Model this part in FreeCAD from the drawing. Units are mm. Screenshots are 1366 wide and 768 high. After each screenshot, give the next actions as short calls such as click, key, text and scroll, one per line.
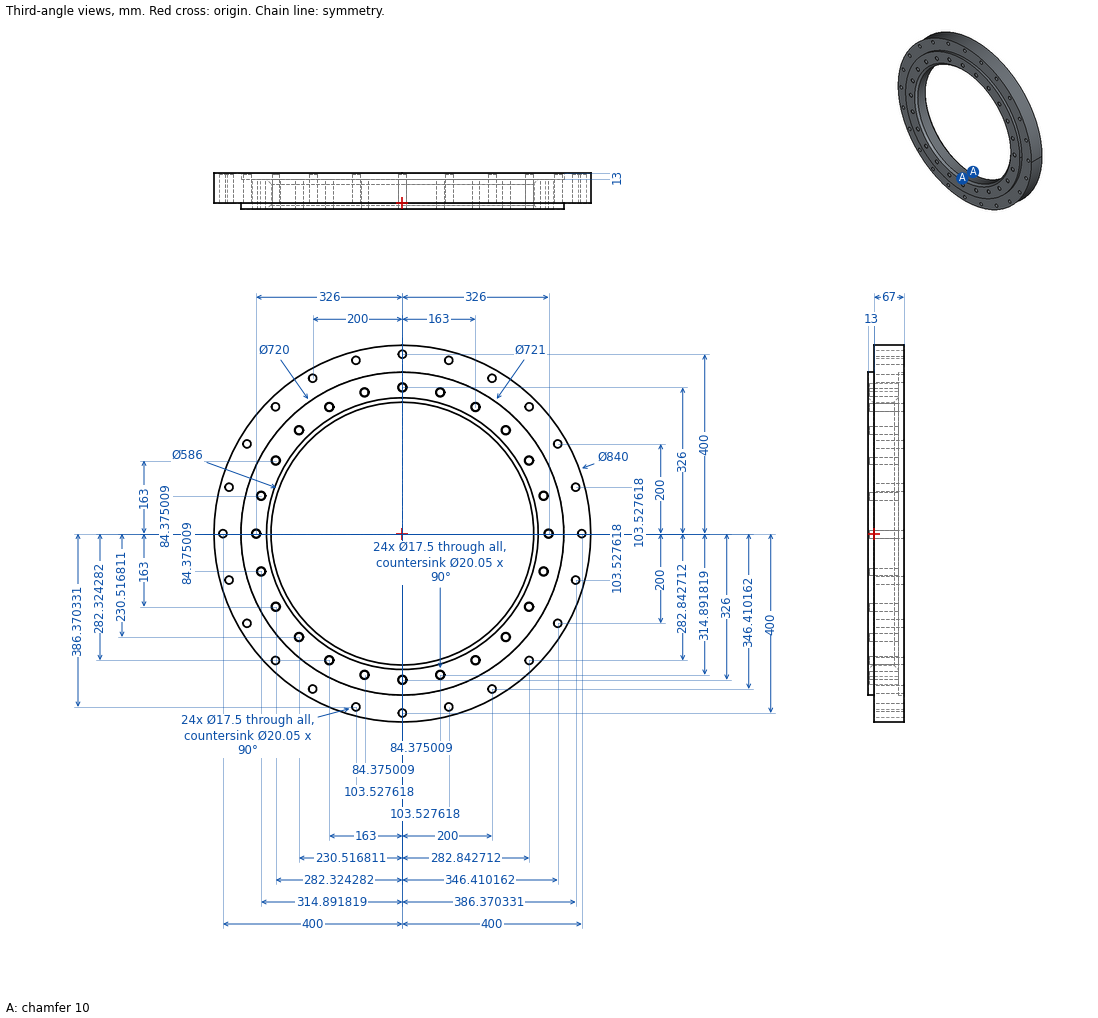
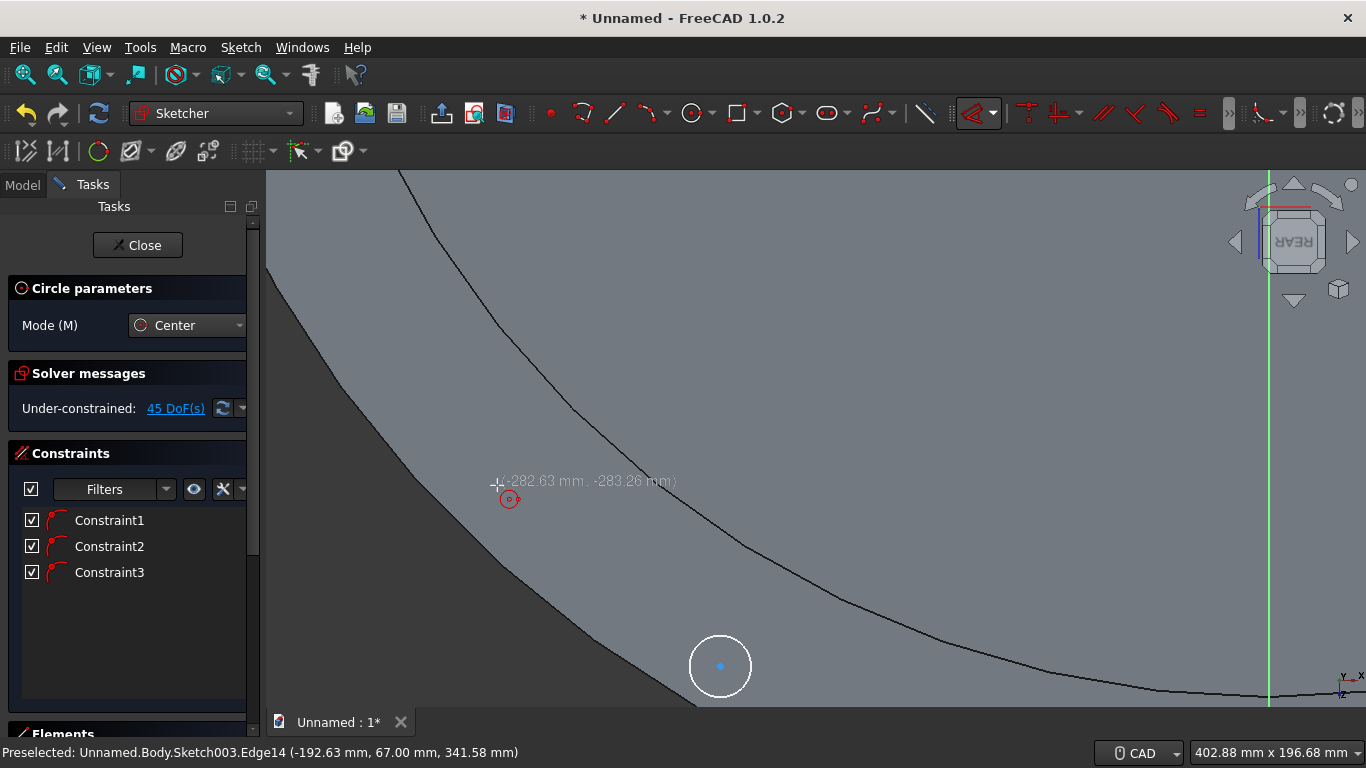
scroll(644, 582, down, 9)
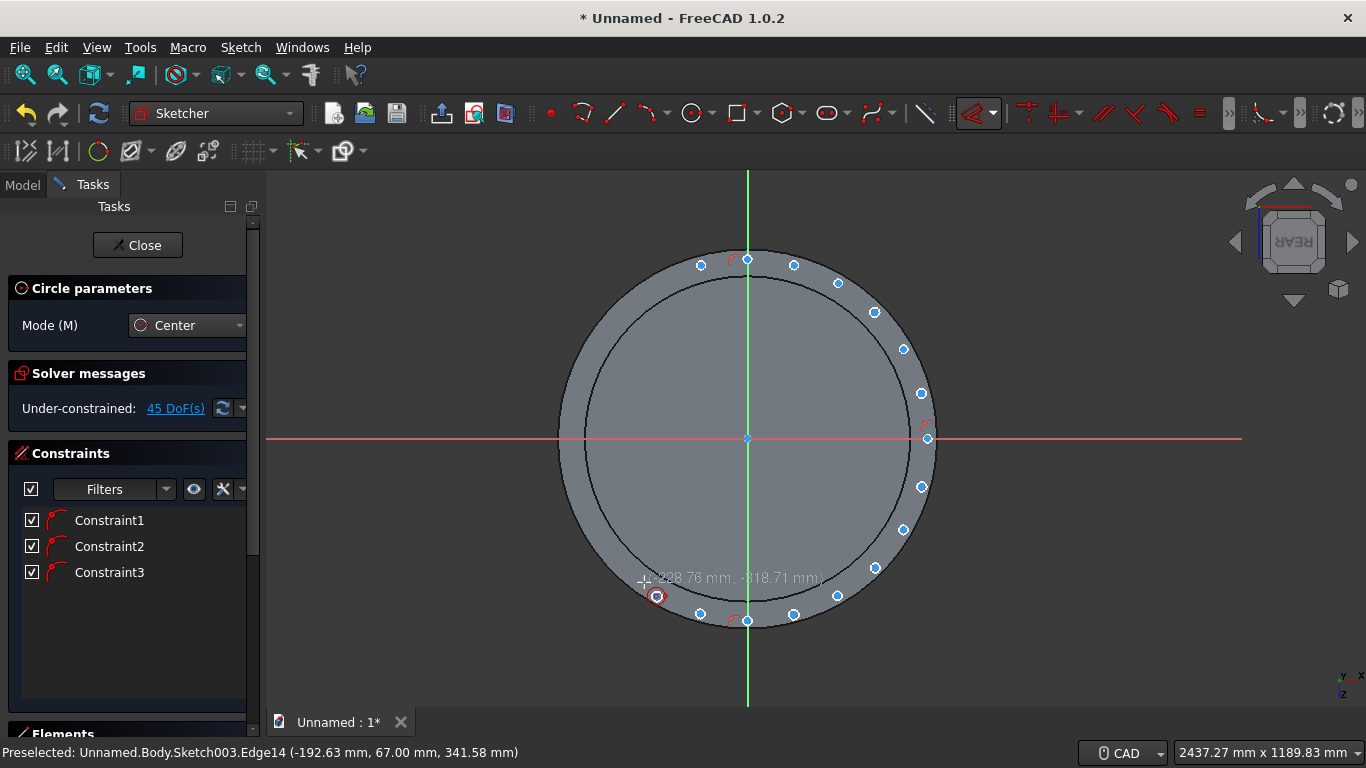
click(620, 567)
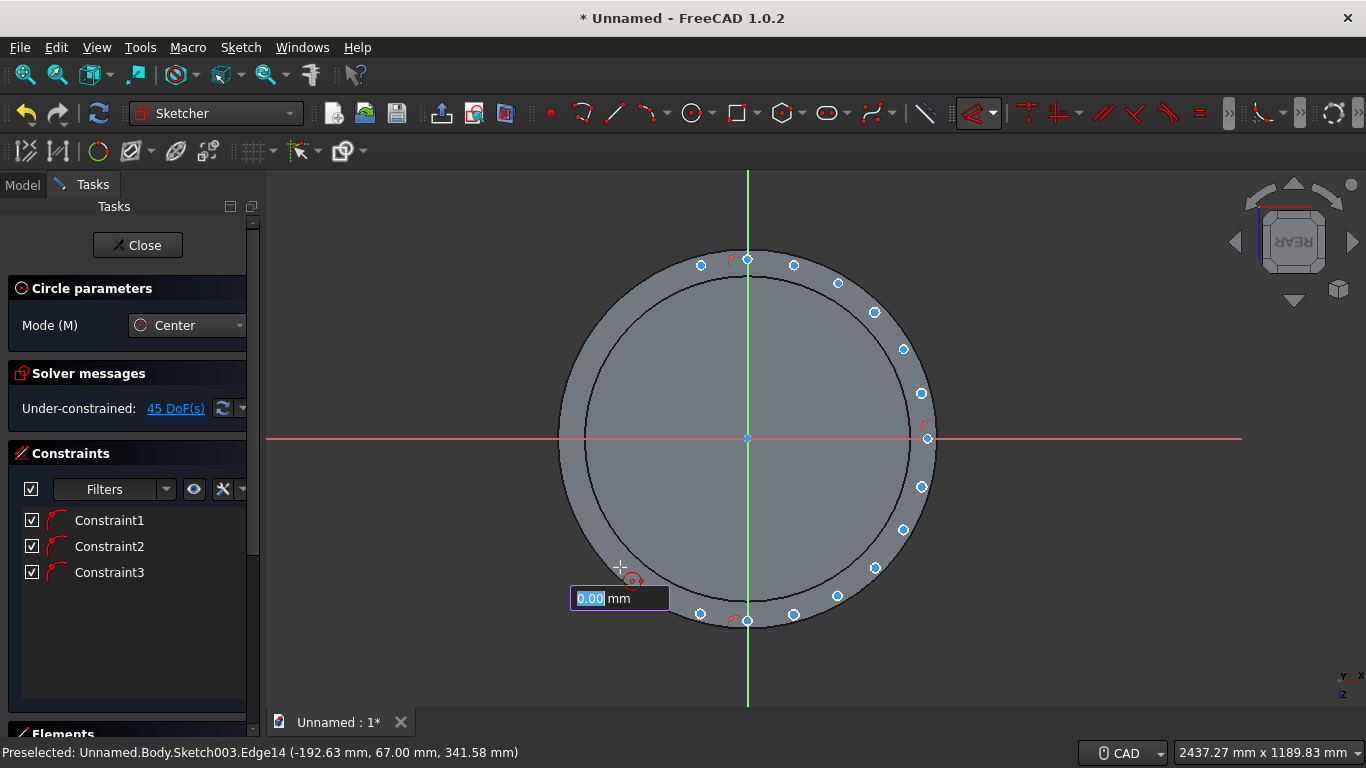
scroll(623, 564, up, 7)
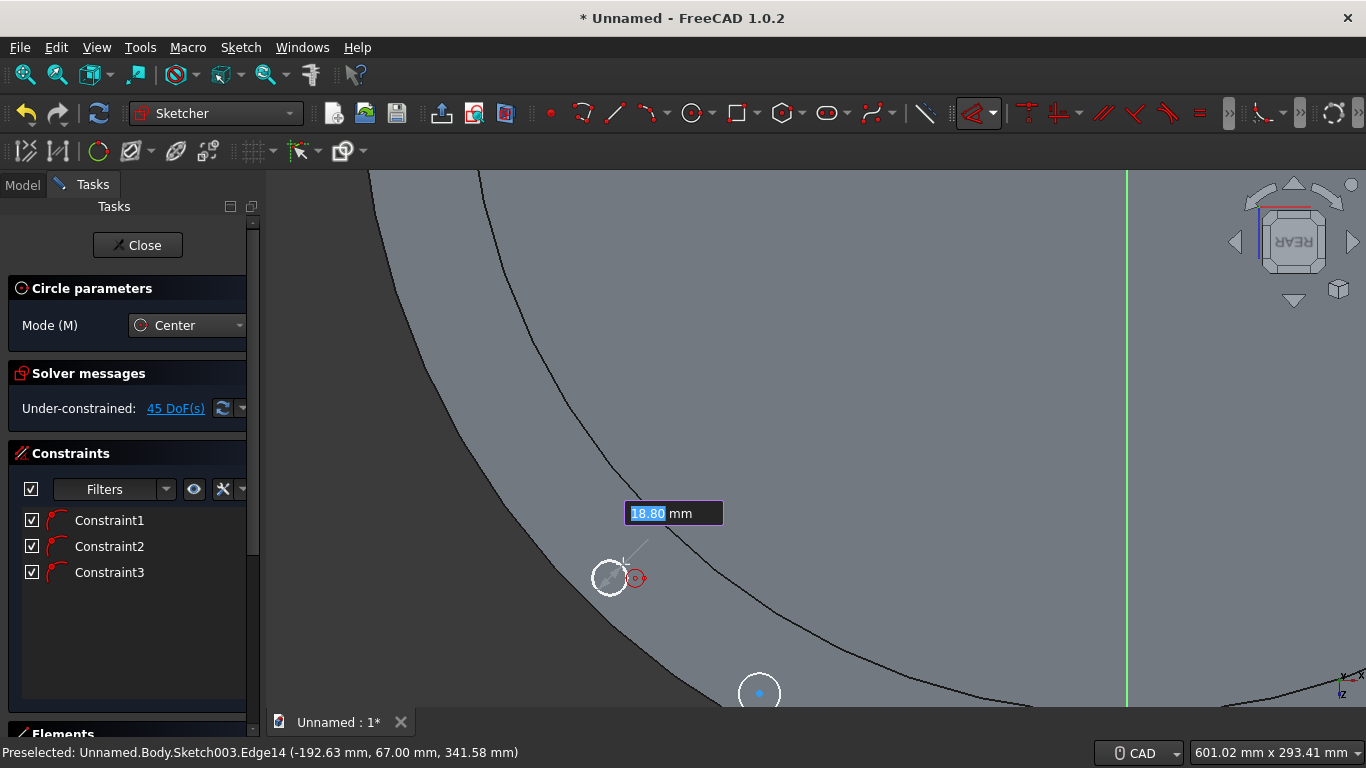
click(621, 561)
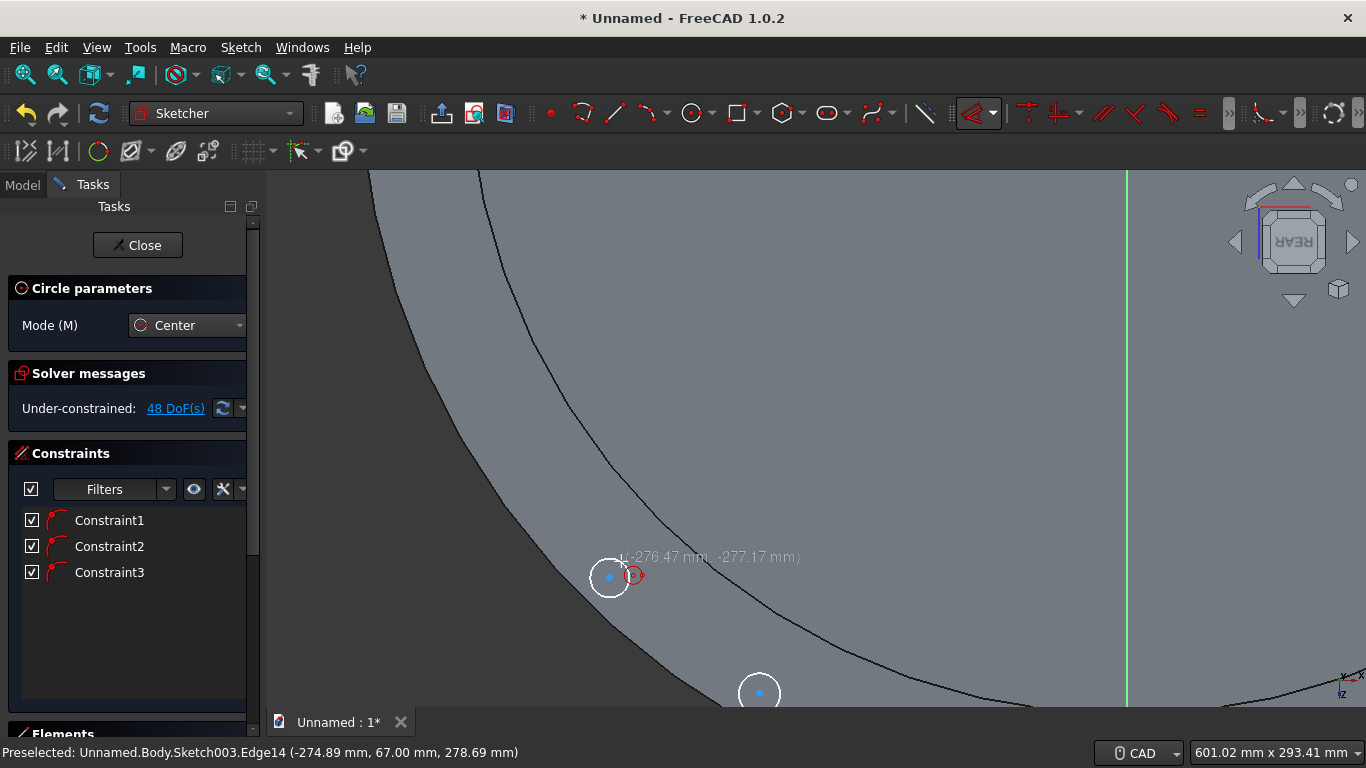
scroll(493, 421, up, 2)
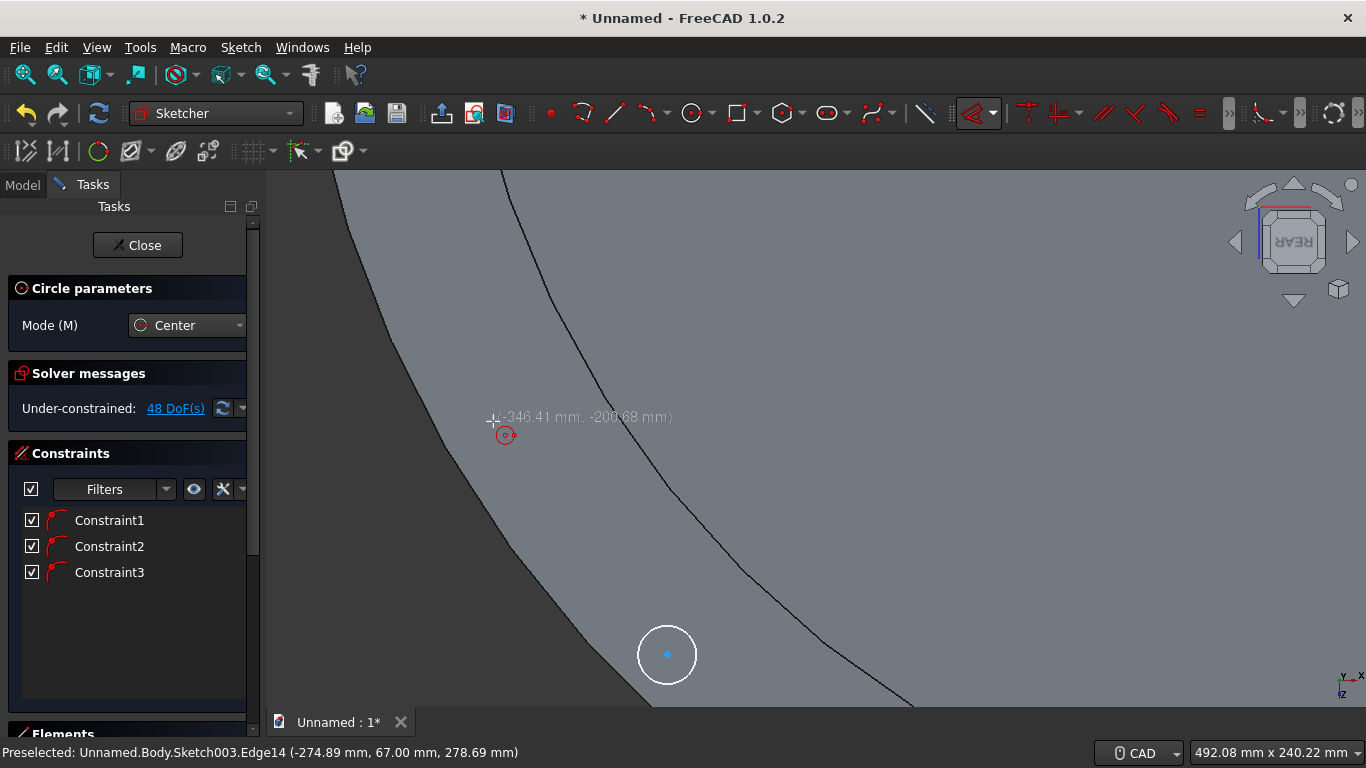
scroll(611, 550, down, 9)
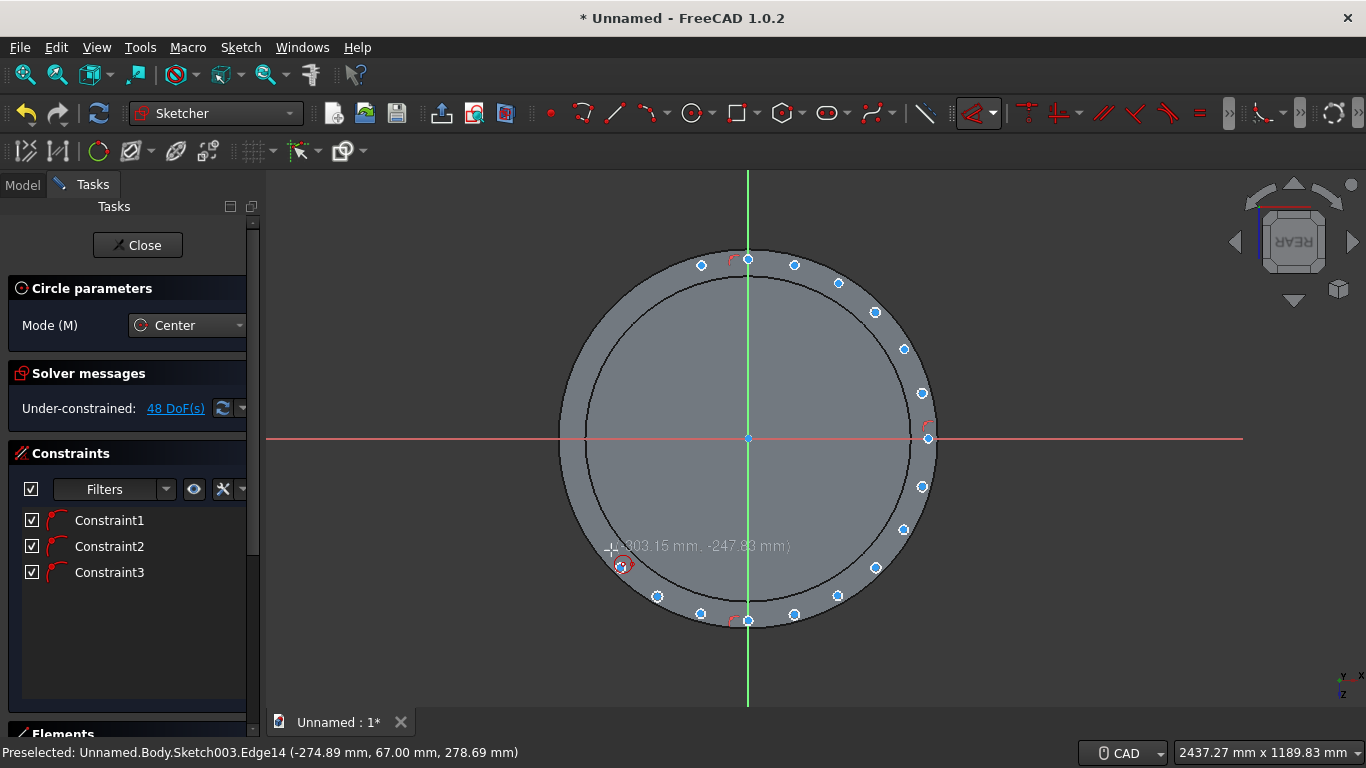
click(592, 529)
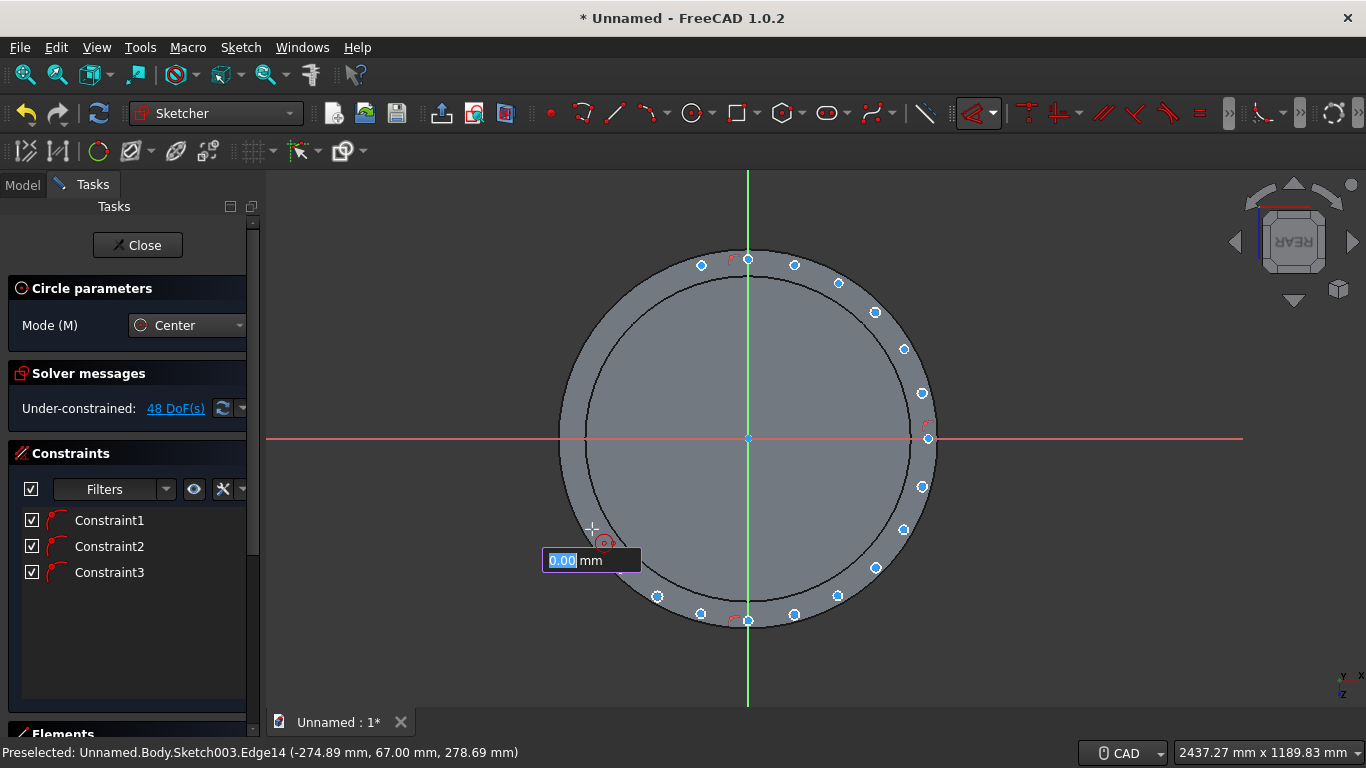
scroll(595, 526, up, 7)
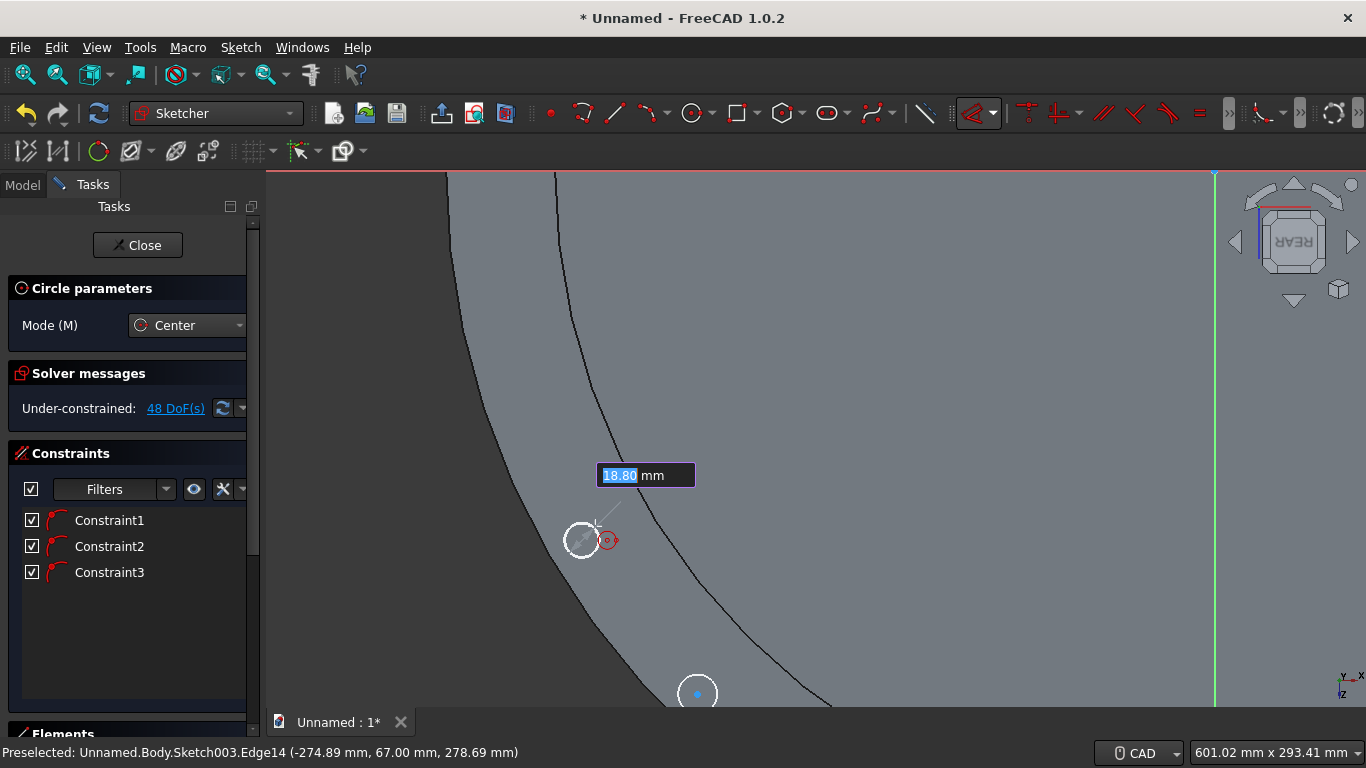
click(592, 526)